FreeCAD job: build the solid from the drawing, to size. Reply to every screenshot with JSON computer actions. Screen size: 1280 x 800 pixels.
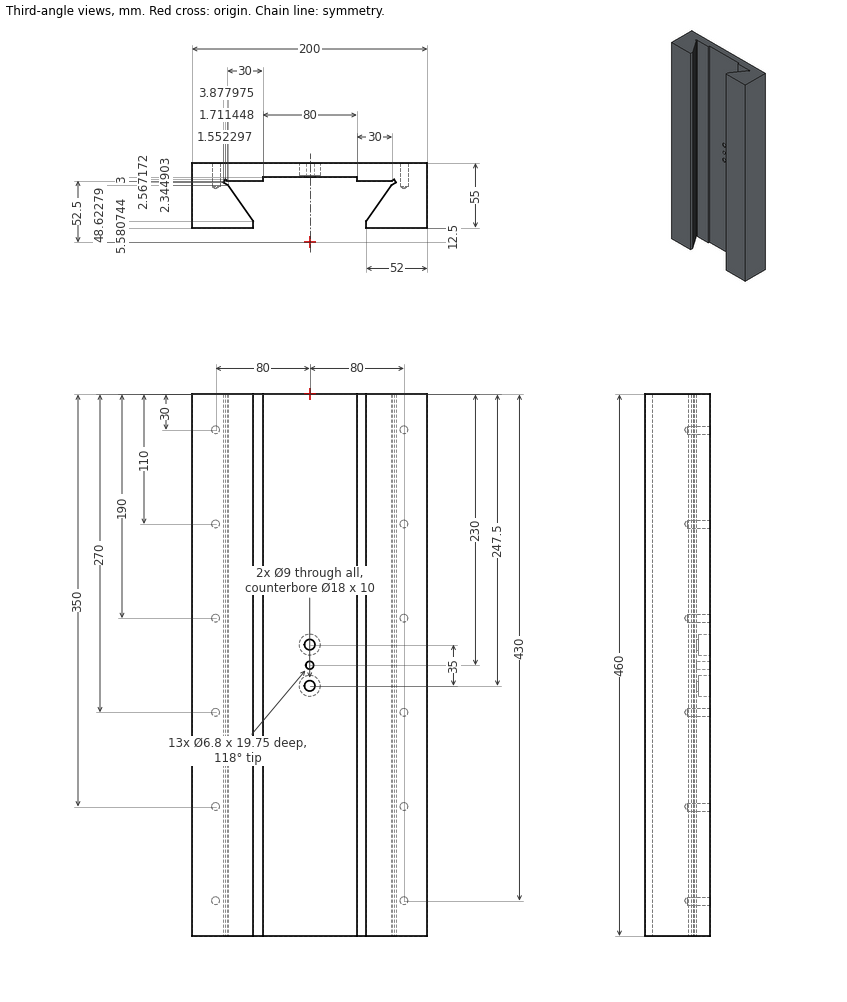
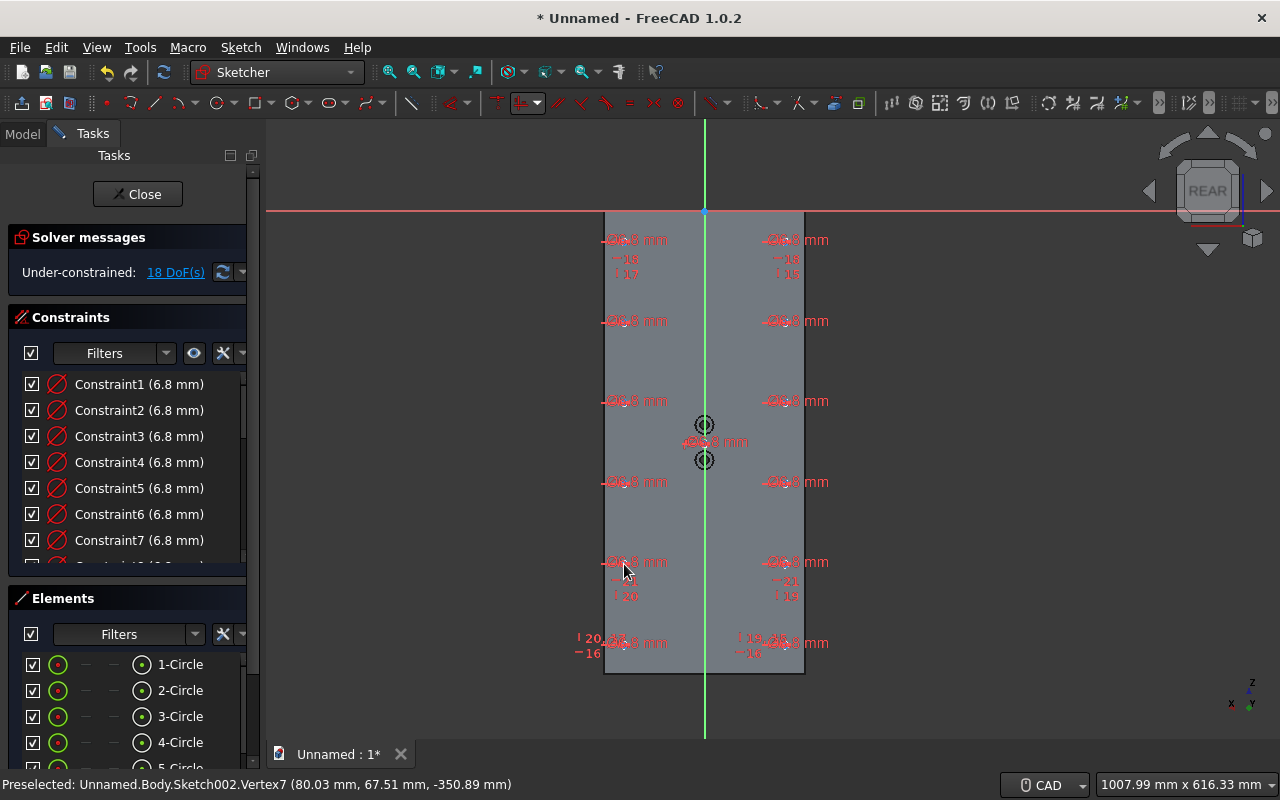
{"action": "left_click", "coordinate": [785, 564]}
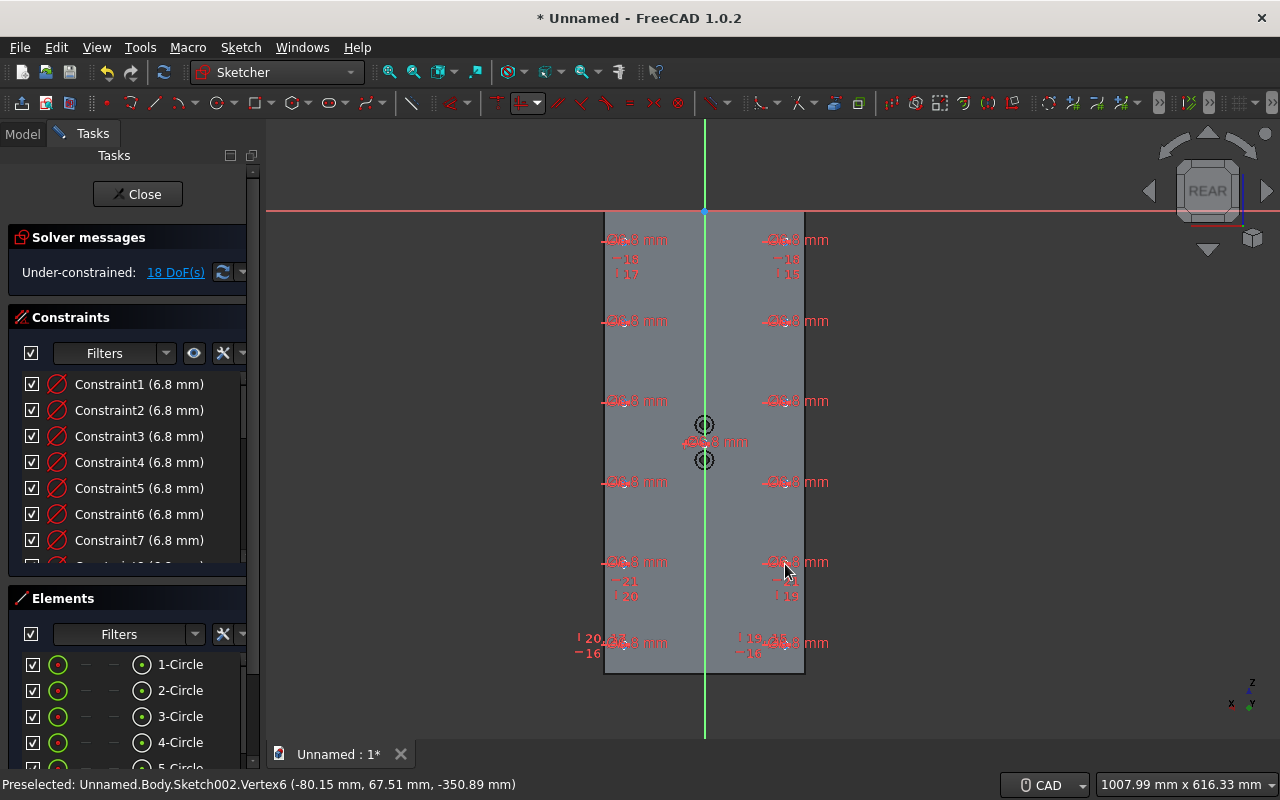
{"action": "left_click", "coordinate": [785, 484]}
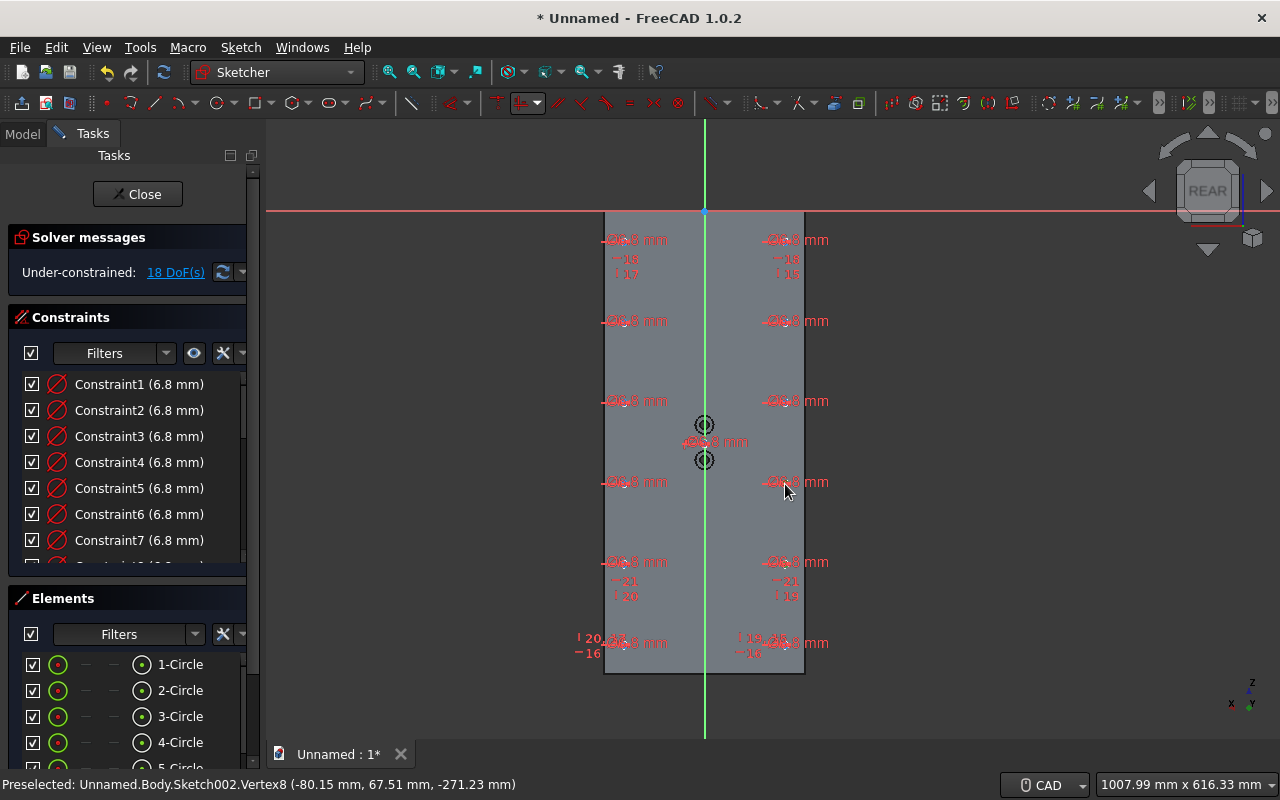
{"action": "key", "text": "v"}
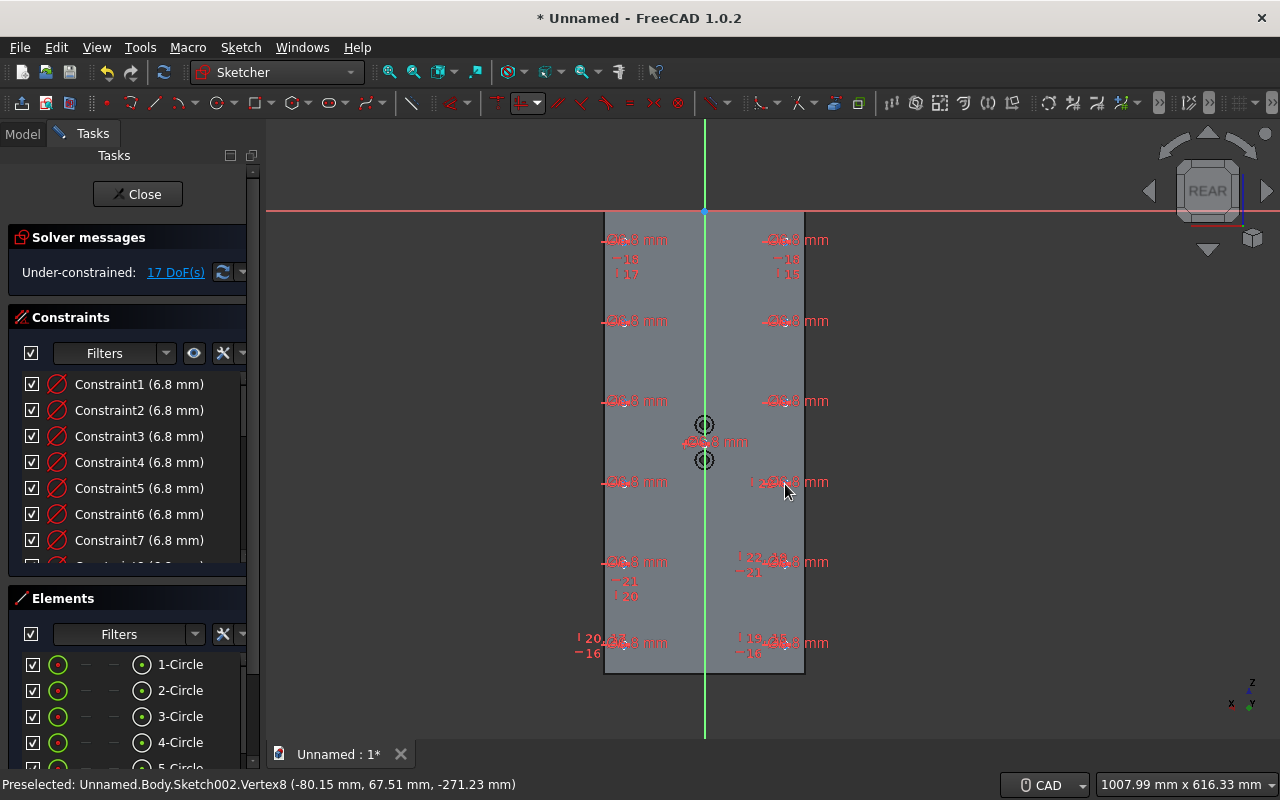
{"action": "left_click", "coordinate": [624, 564]}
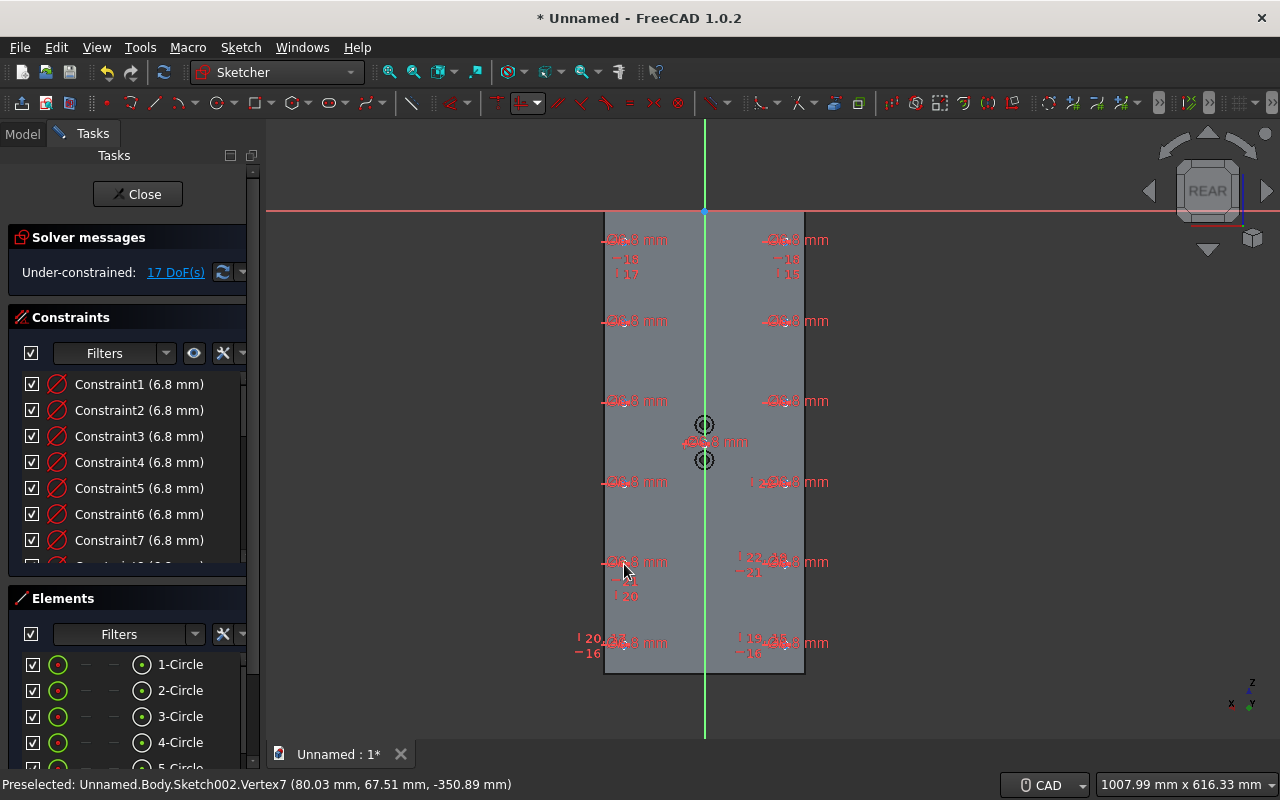
{"action": "left_click", "coordinate": [624, 484]}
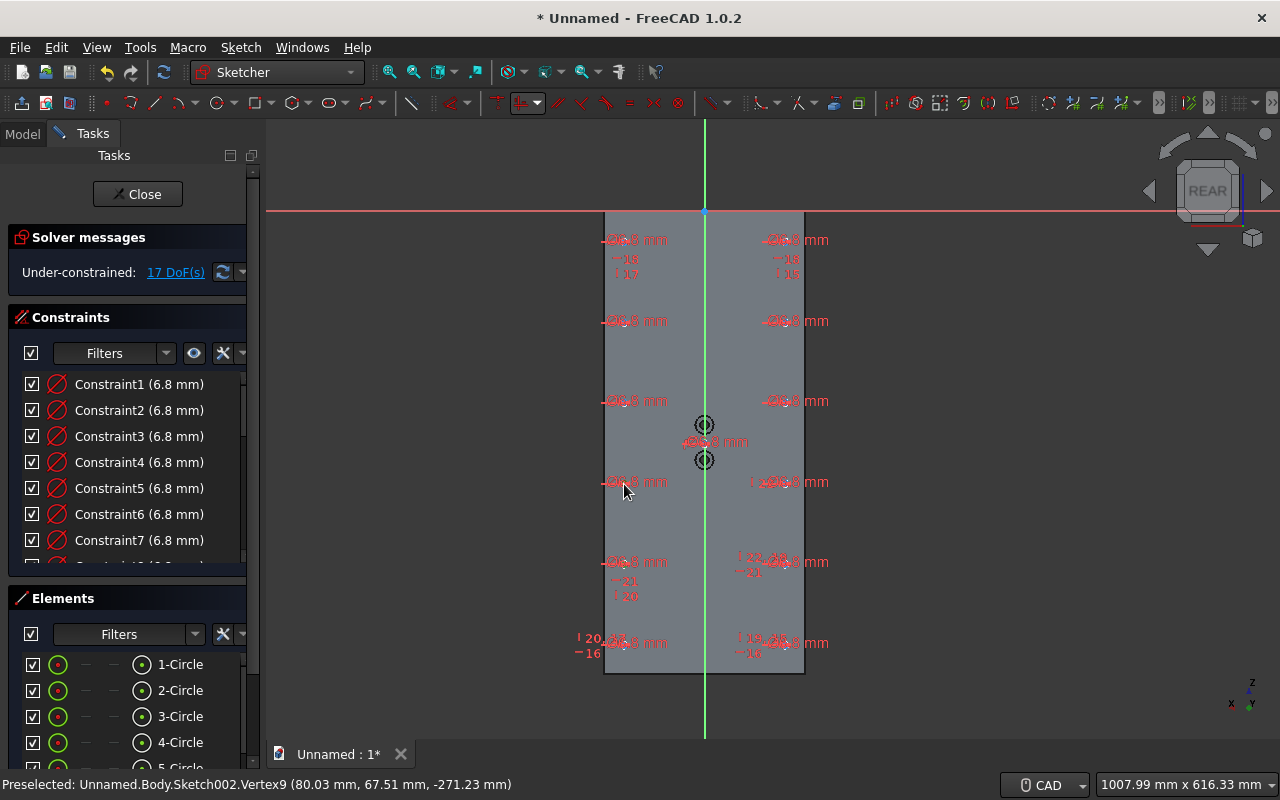
{"action": "key", "text": "v"}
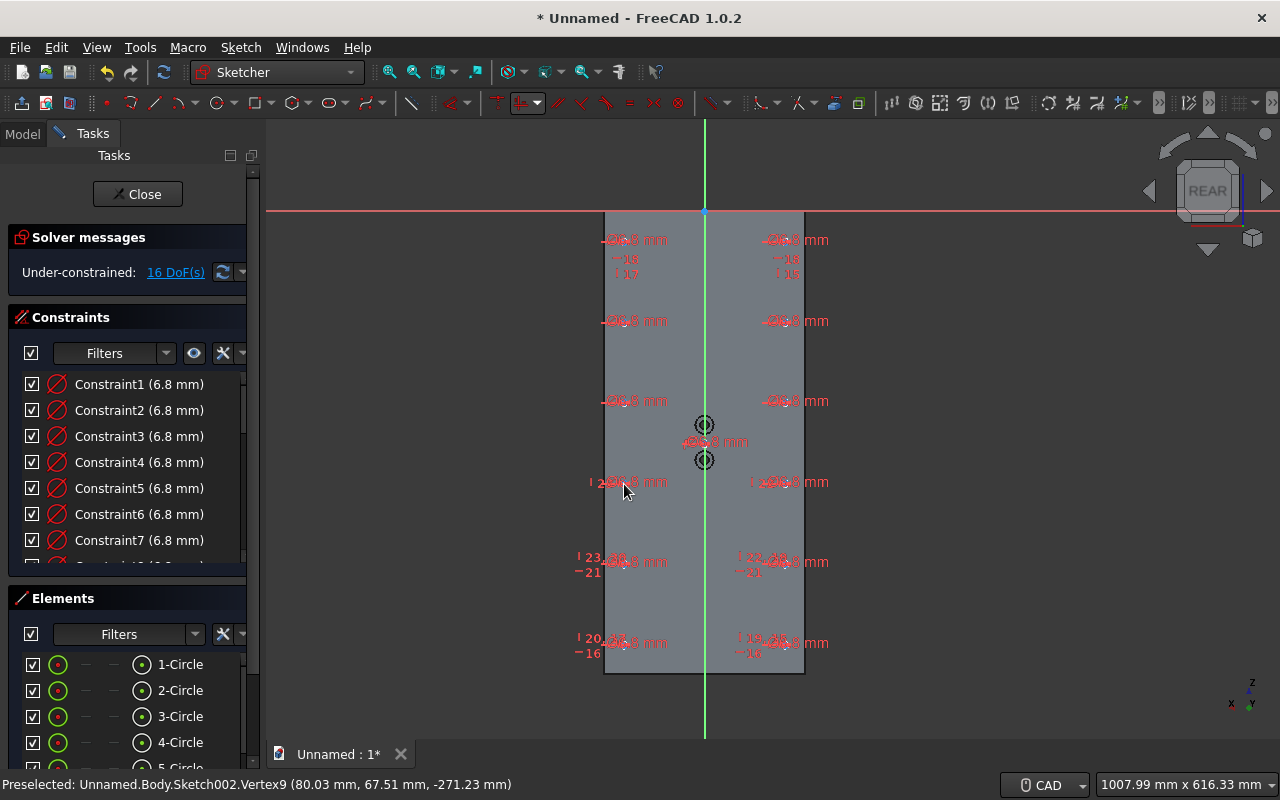
{"action": "left_click", "coordinate": [785, 484]}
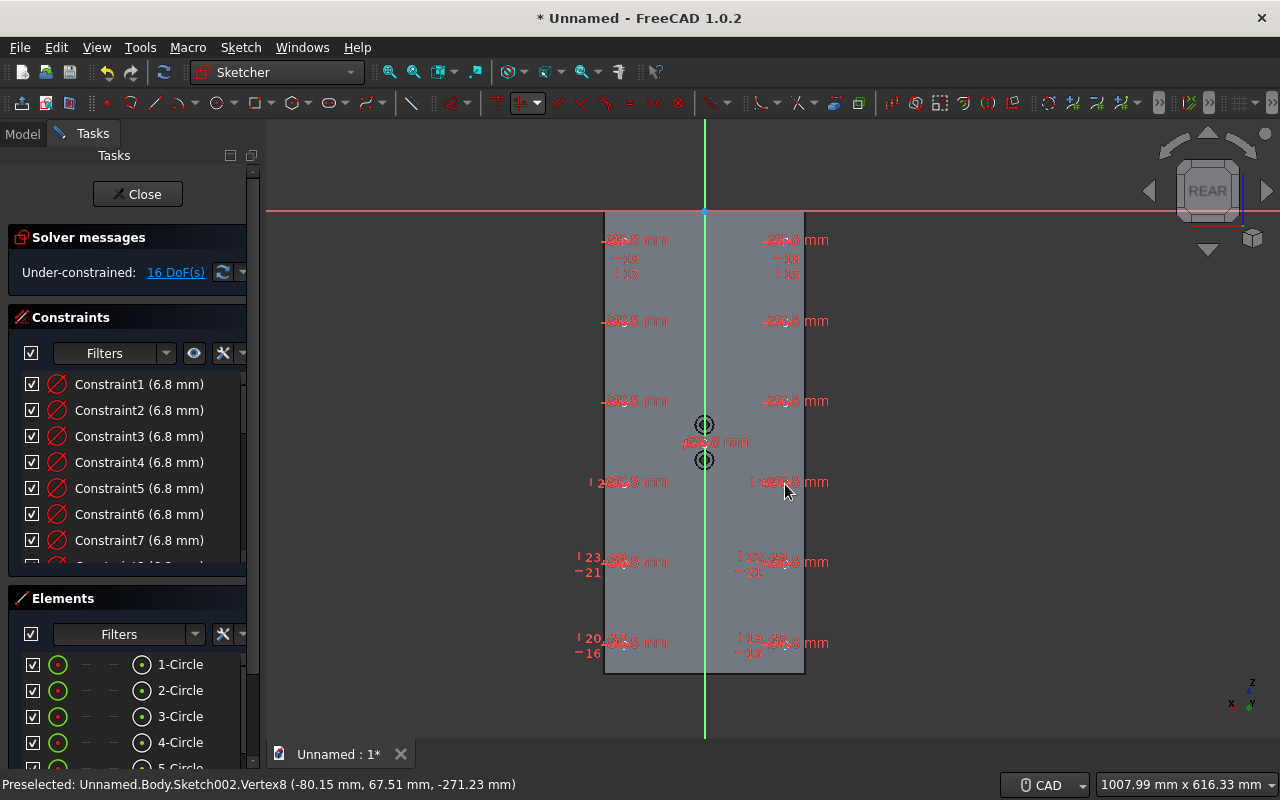
{"action": "left_click", "coordinate": [624, 484]}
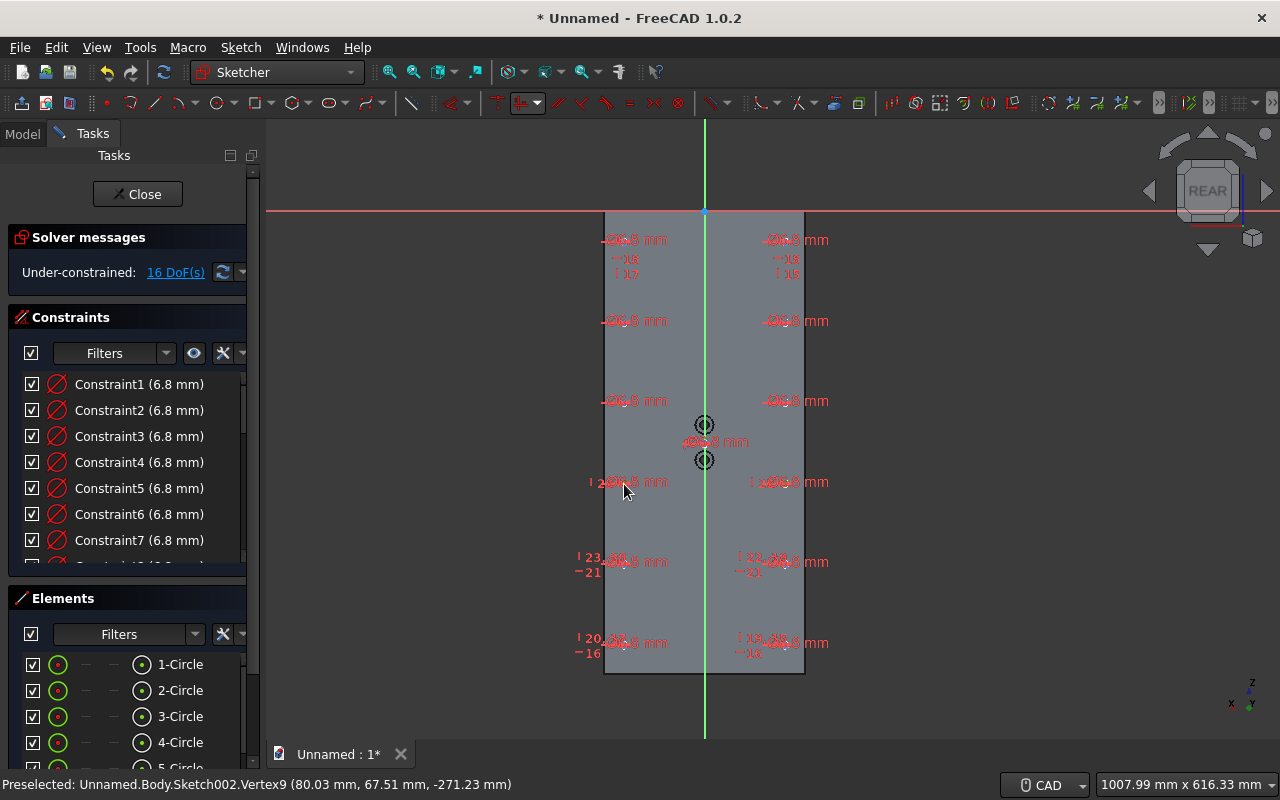
{"action": "left_click", "coordinate": [540, 104]}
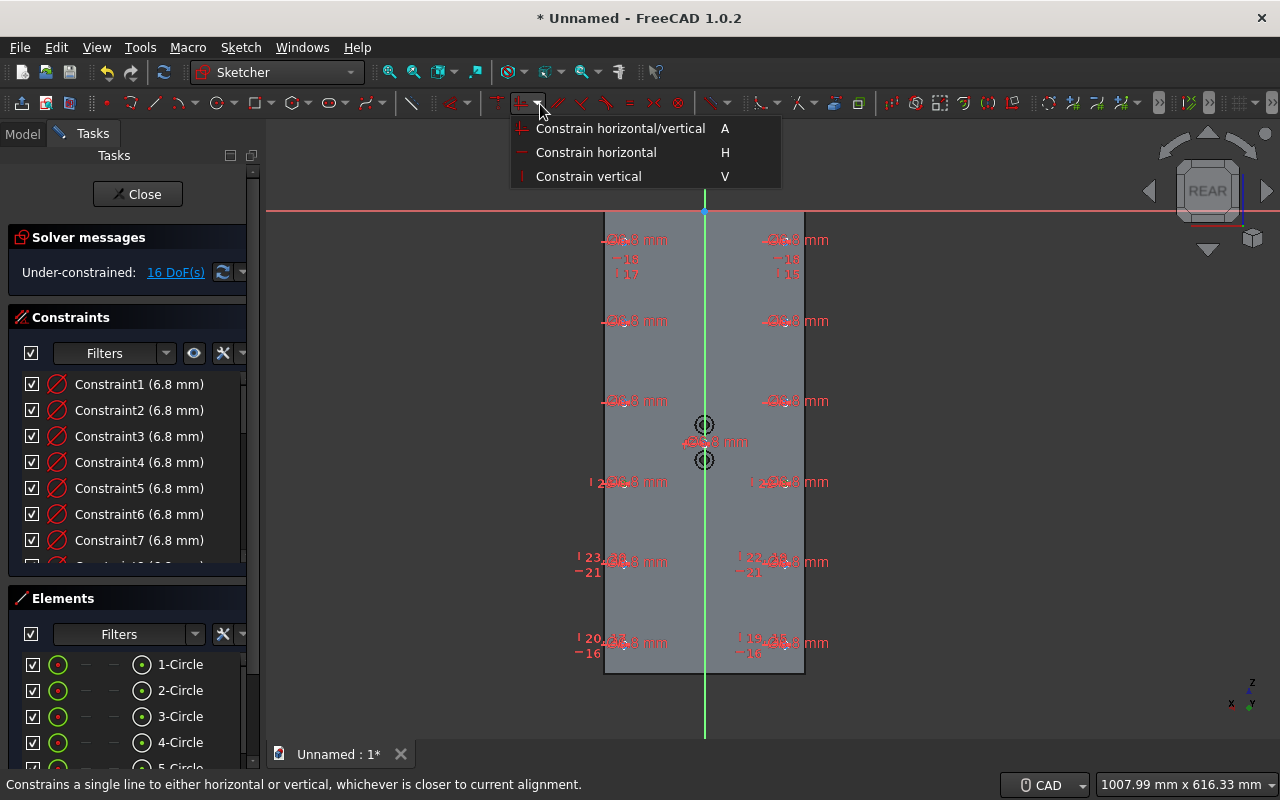
{"action": "left_click", "coordinate": [646, 152]}